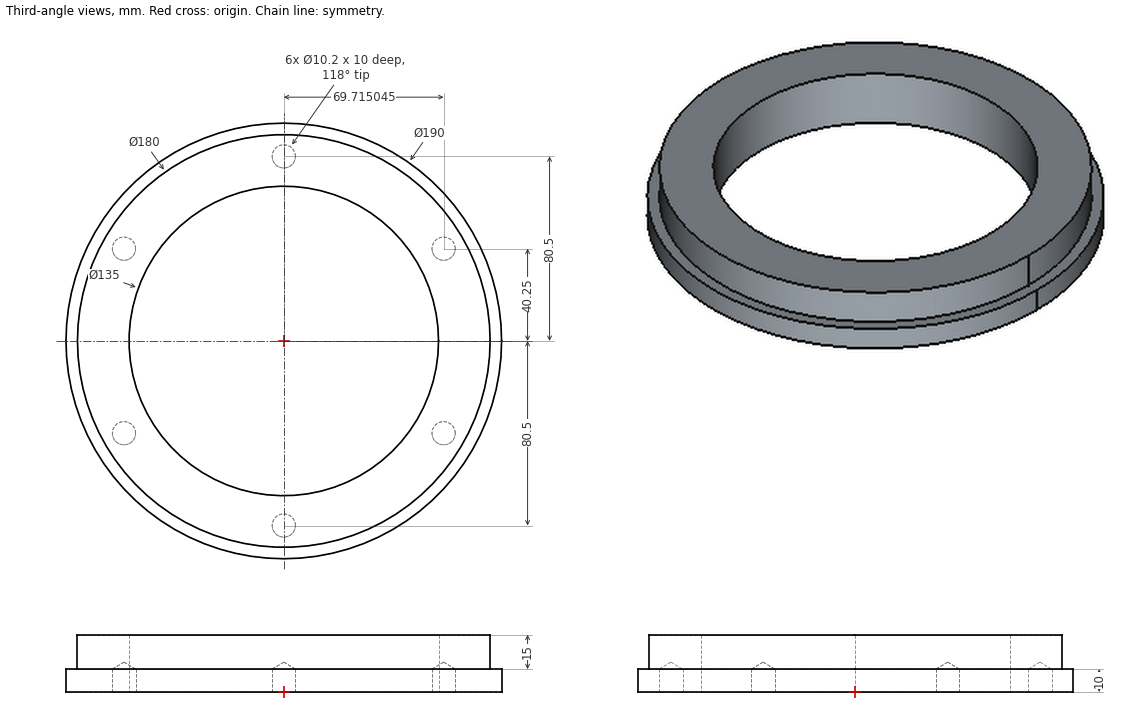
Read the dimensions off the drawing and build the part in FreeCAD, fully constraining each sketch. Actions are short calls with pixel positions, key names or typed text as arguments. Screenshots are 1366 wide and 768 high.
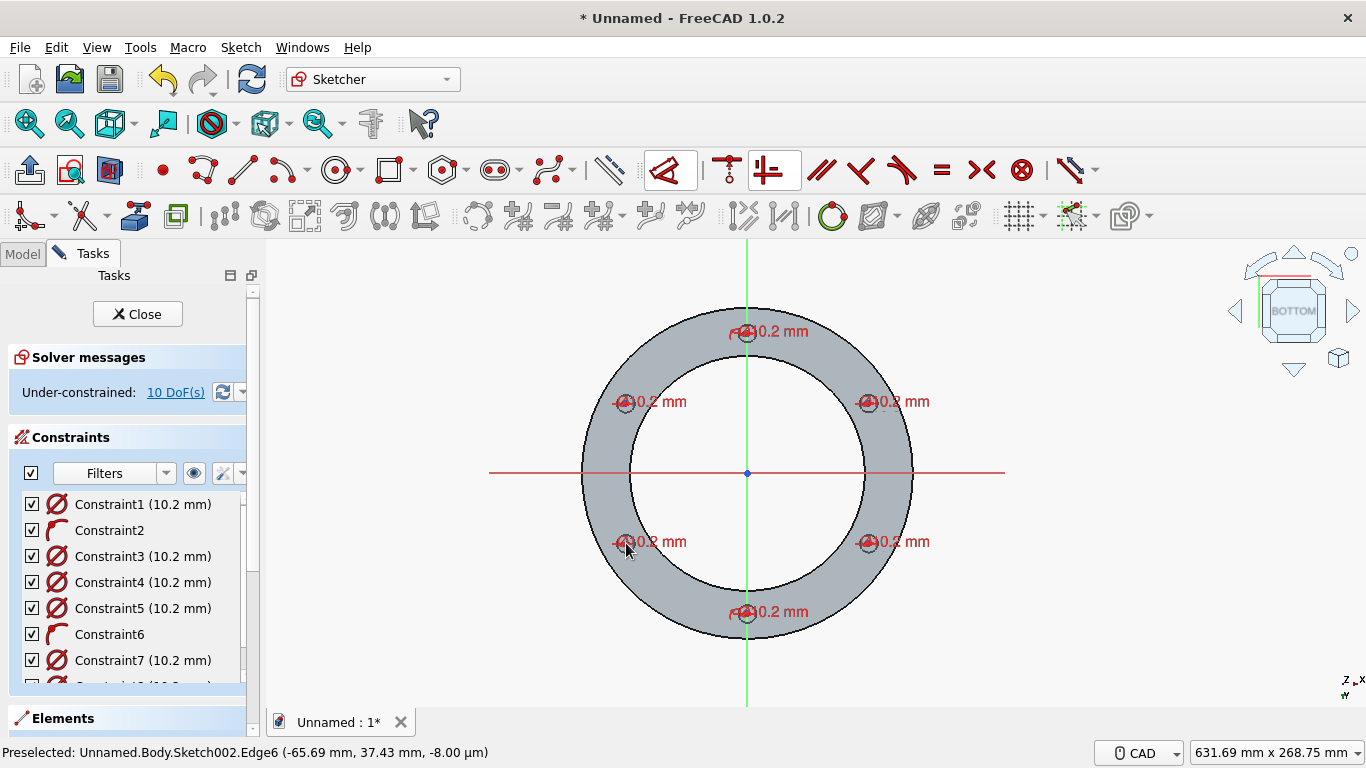
click(869, 544)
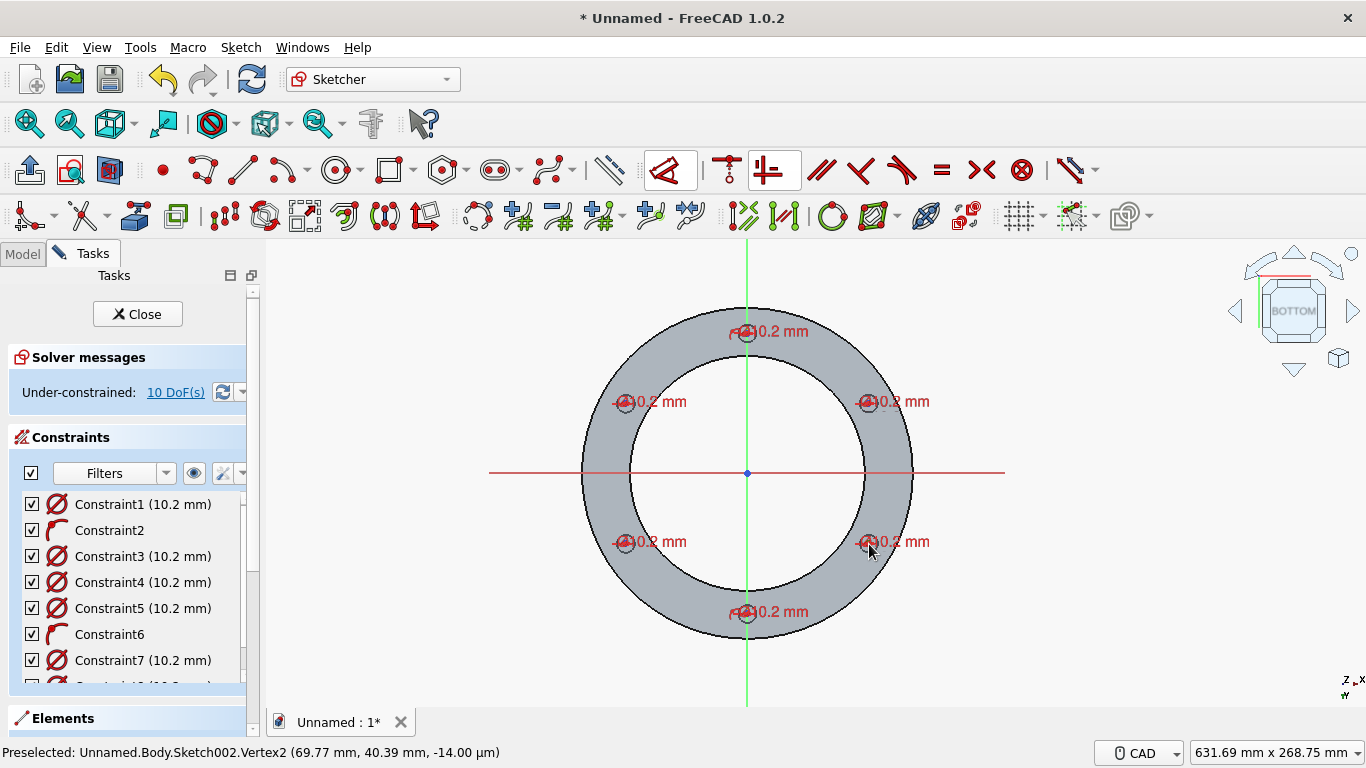
click(869, 404)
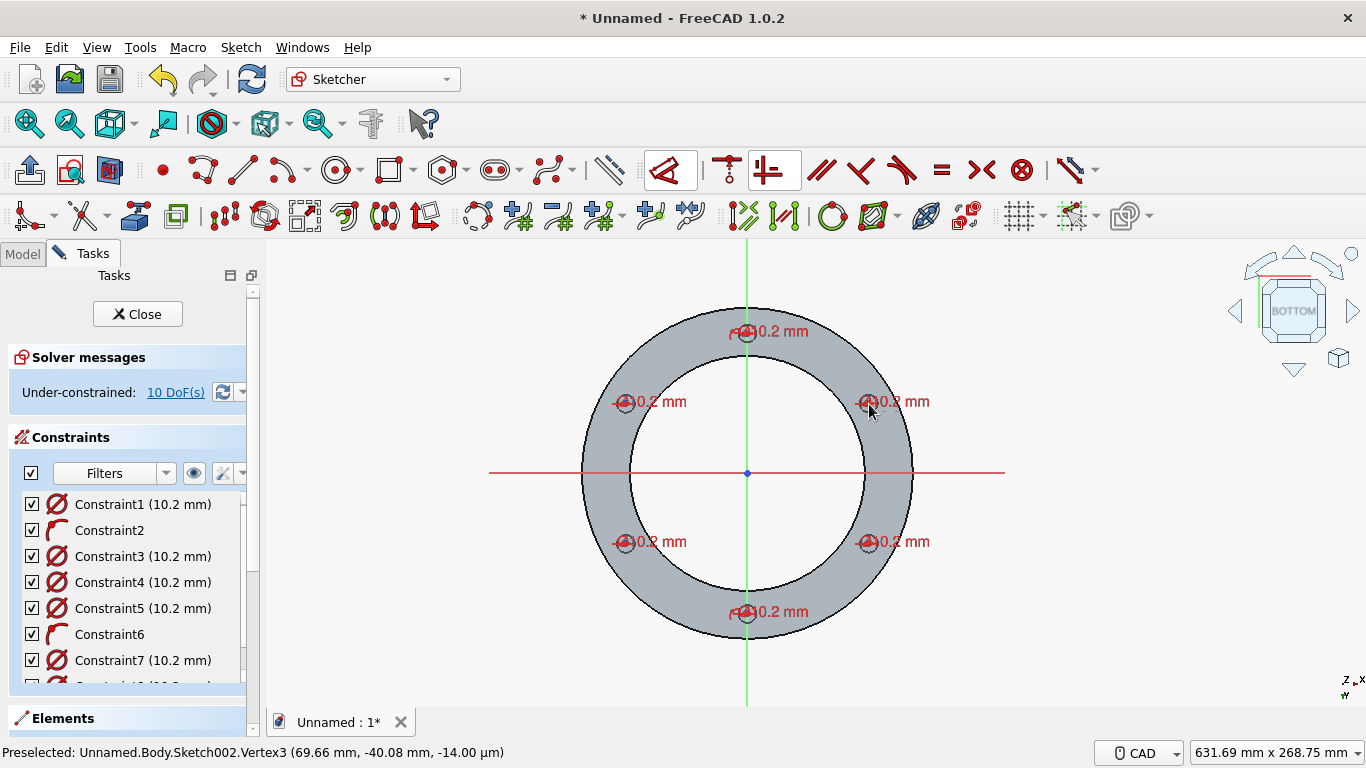
click(488, 473)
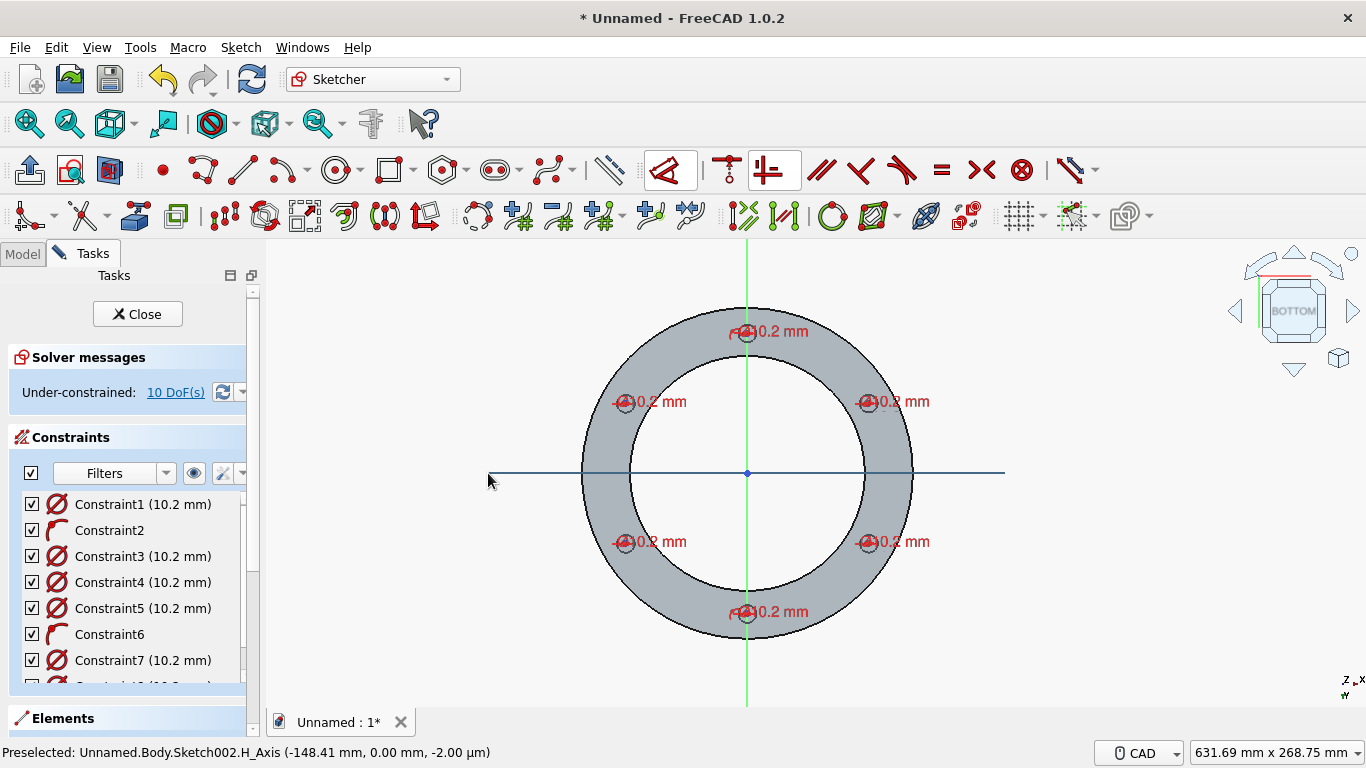
key(s)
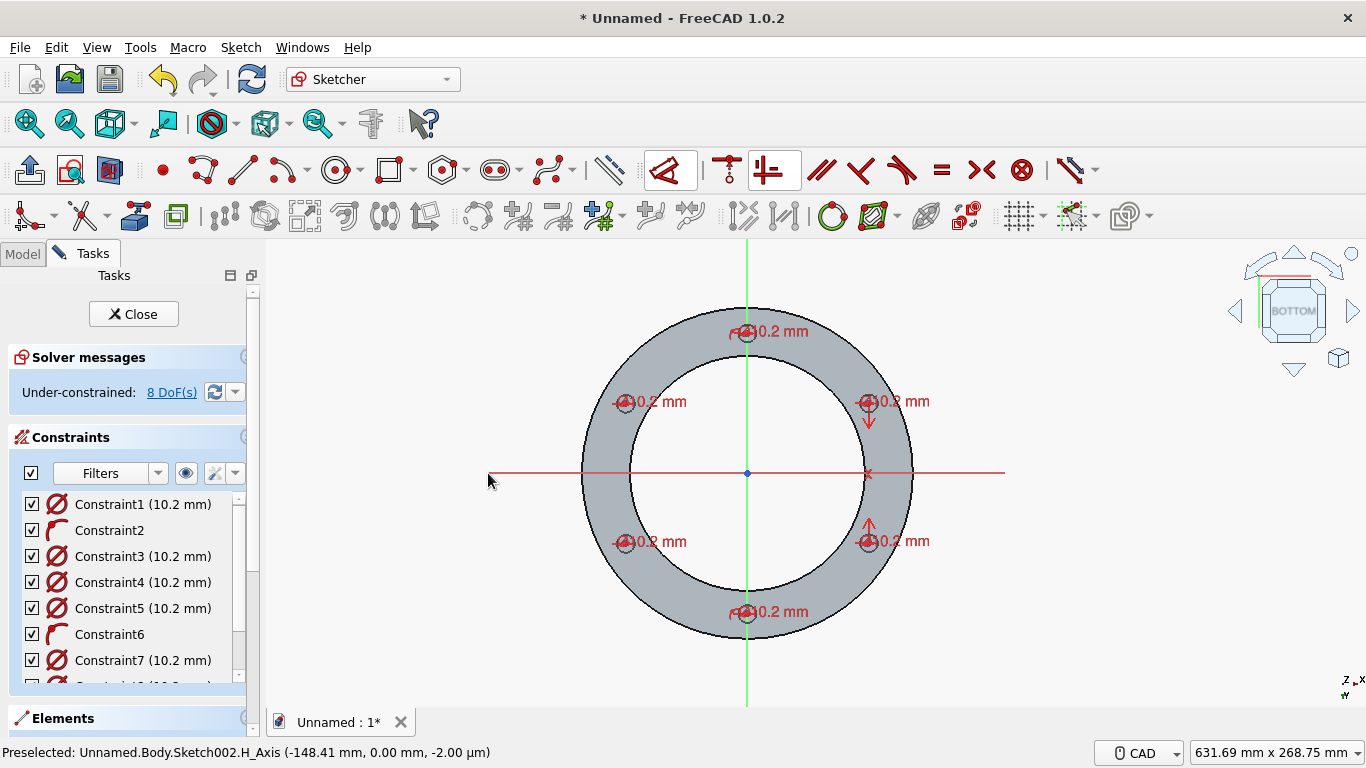
click(869, 403)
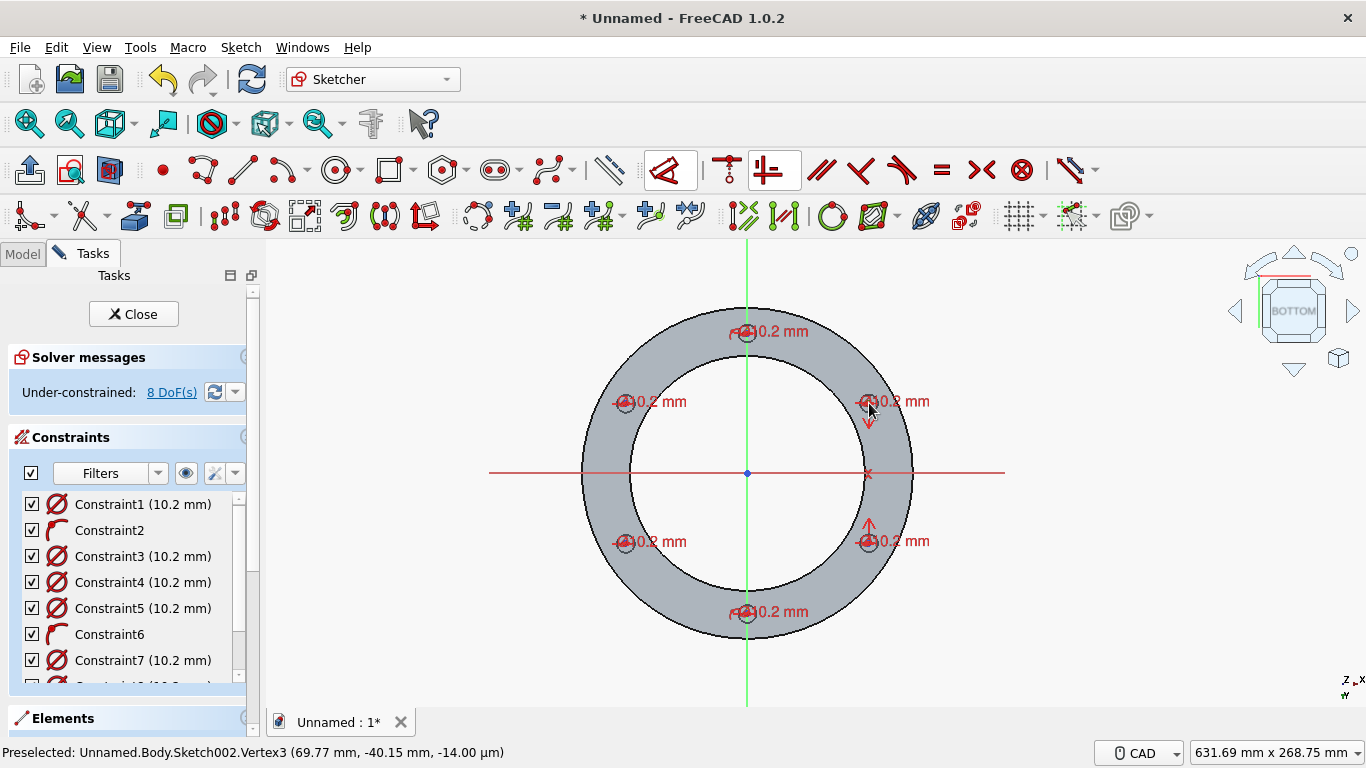
click(626, 404)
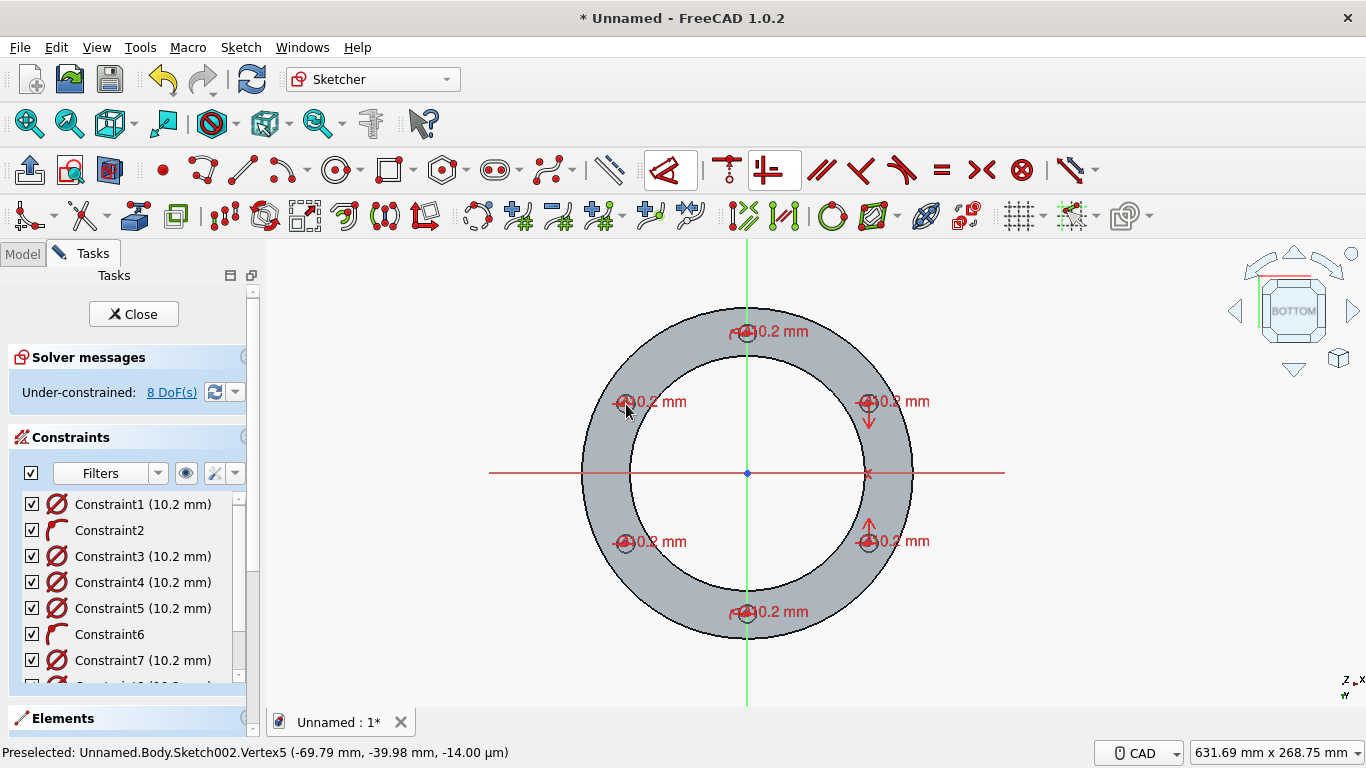
click(747, 561)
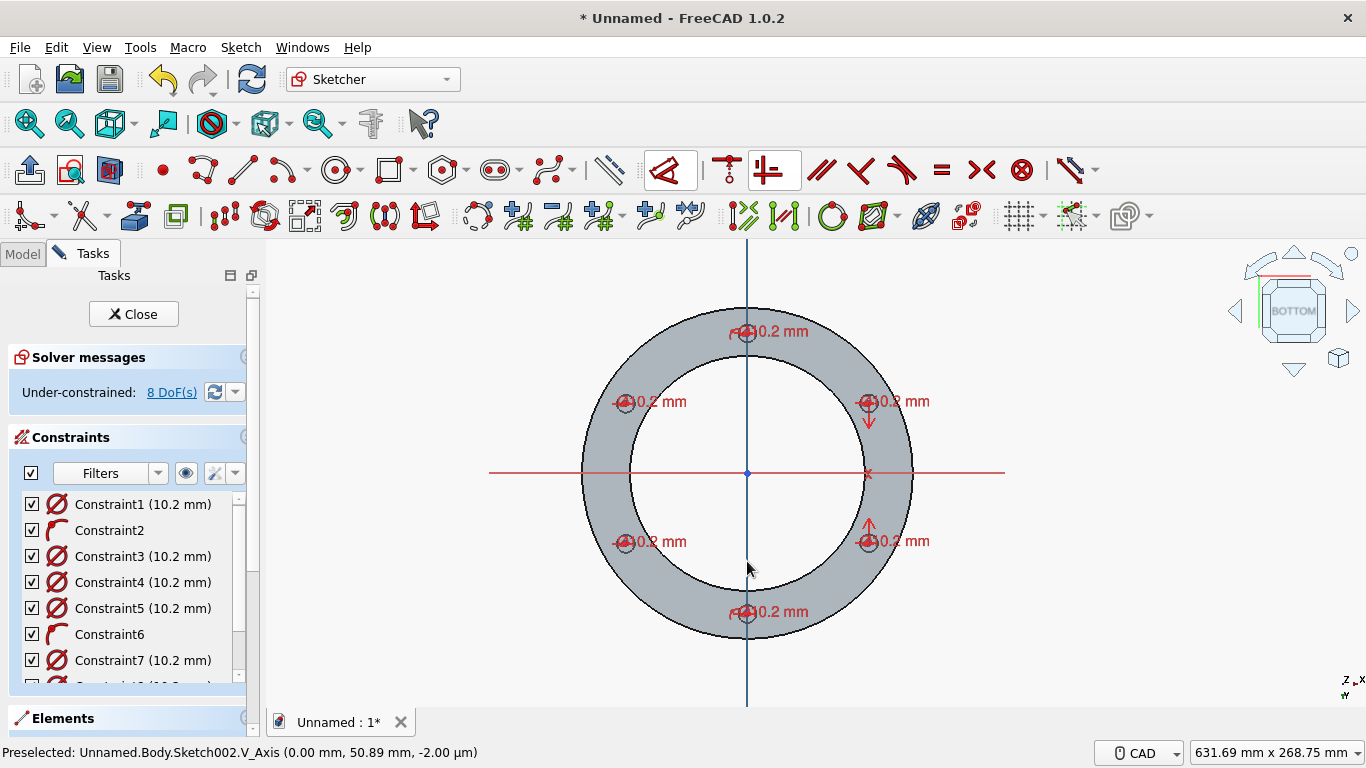
key(s)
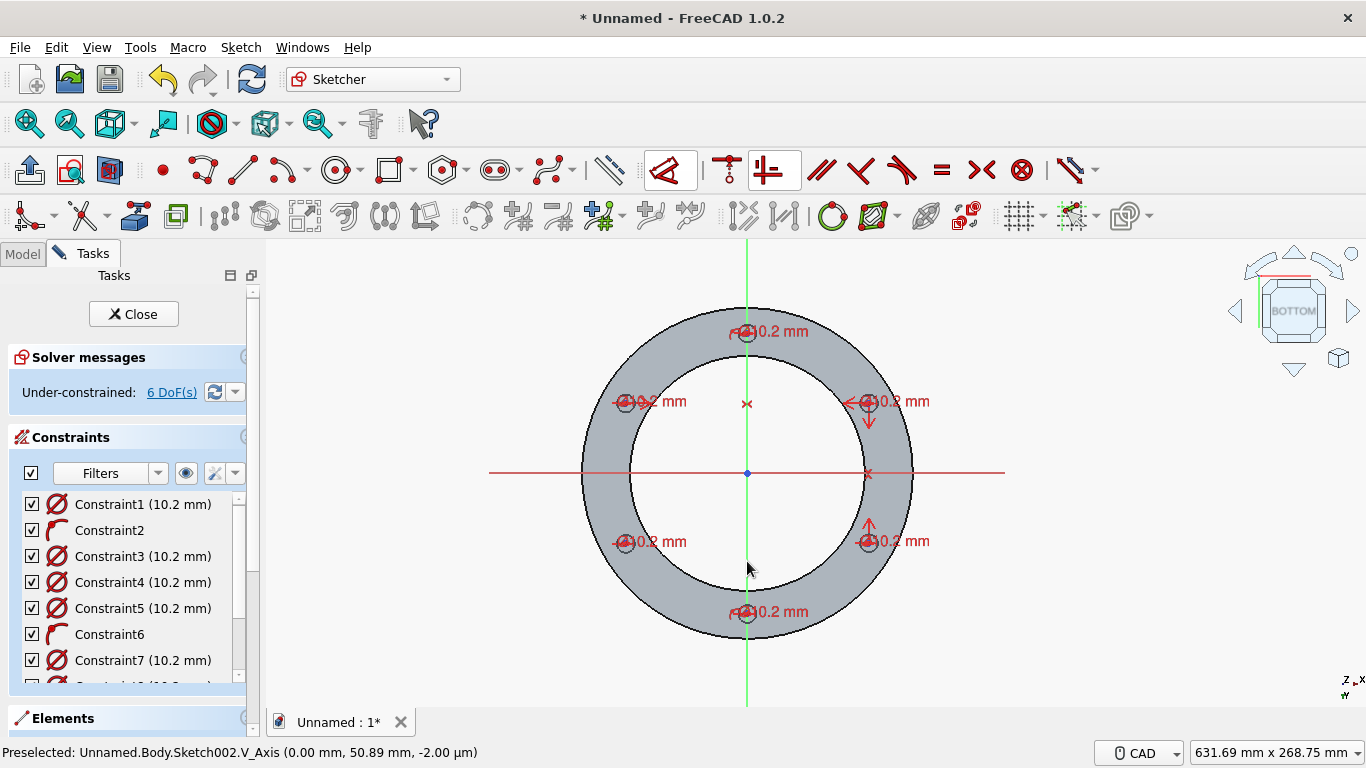
click(869, 543)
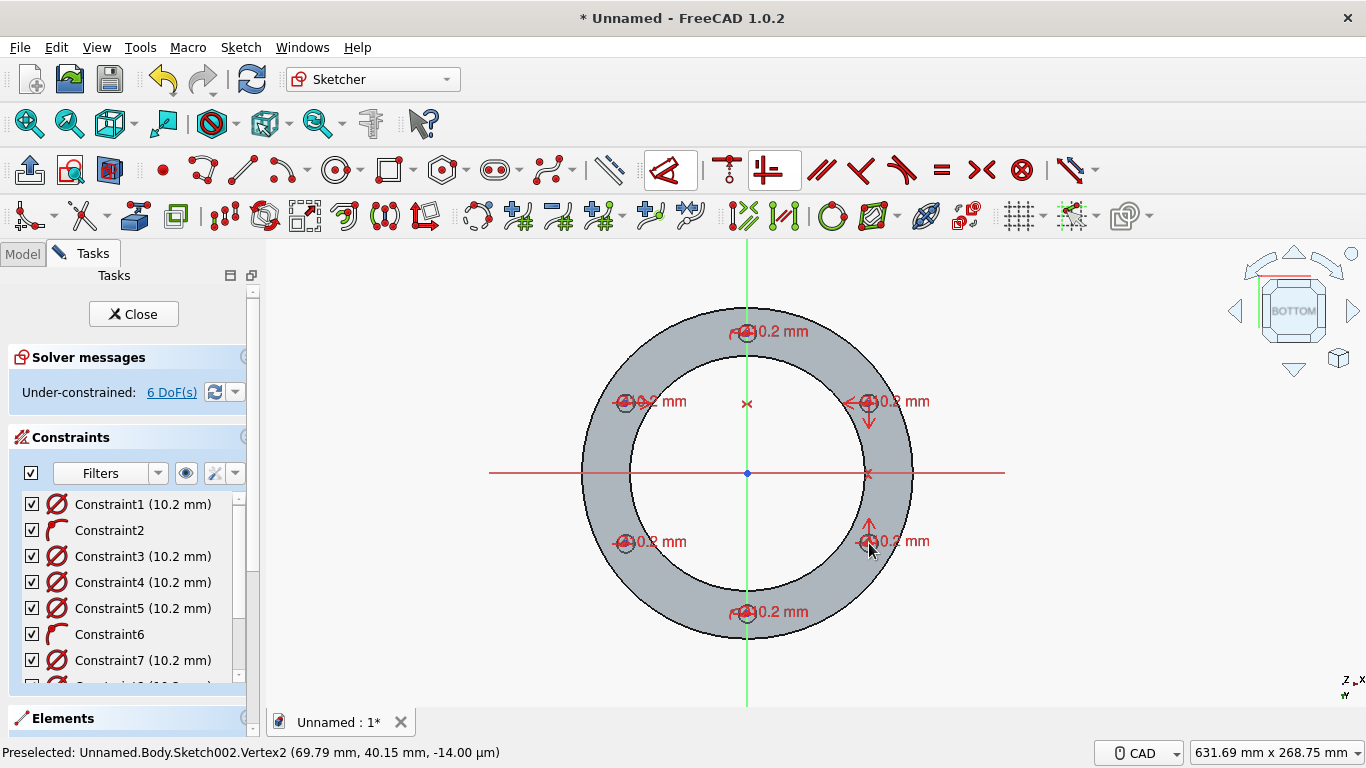
click(626, 544)